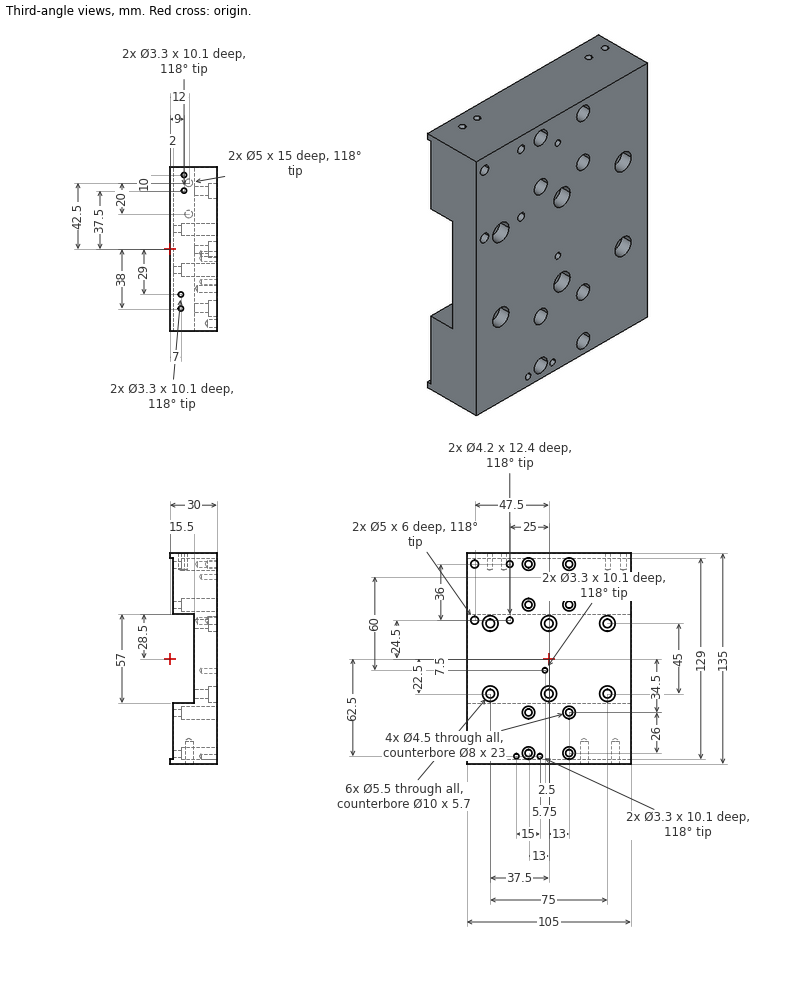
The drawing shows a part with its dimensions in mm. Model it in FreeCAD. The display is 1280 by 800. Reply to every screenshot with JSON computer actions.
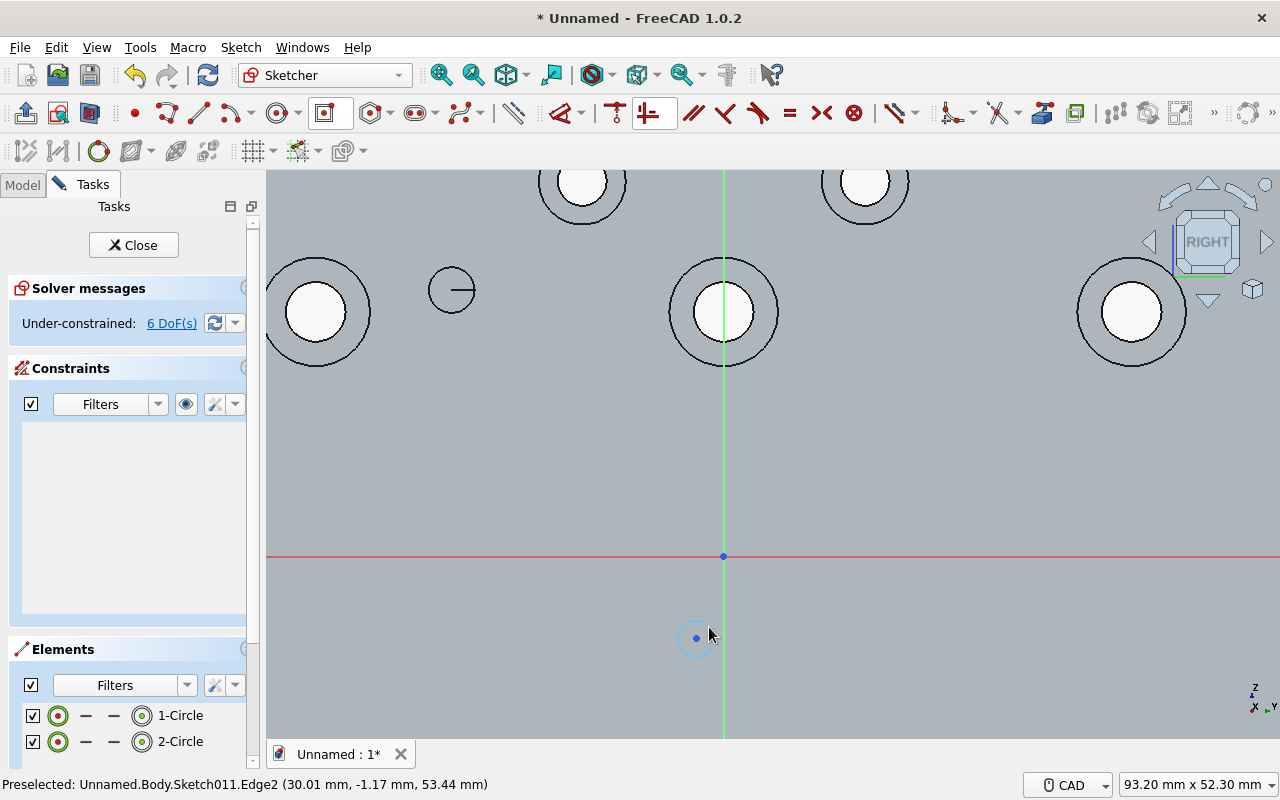
{"action": "left_click", "coordinate": [709, 626]}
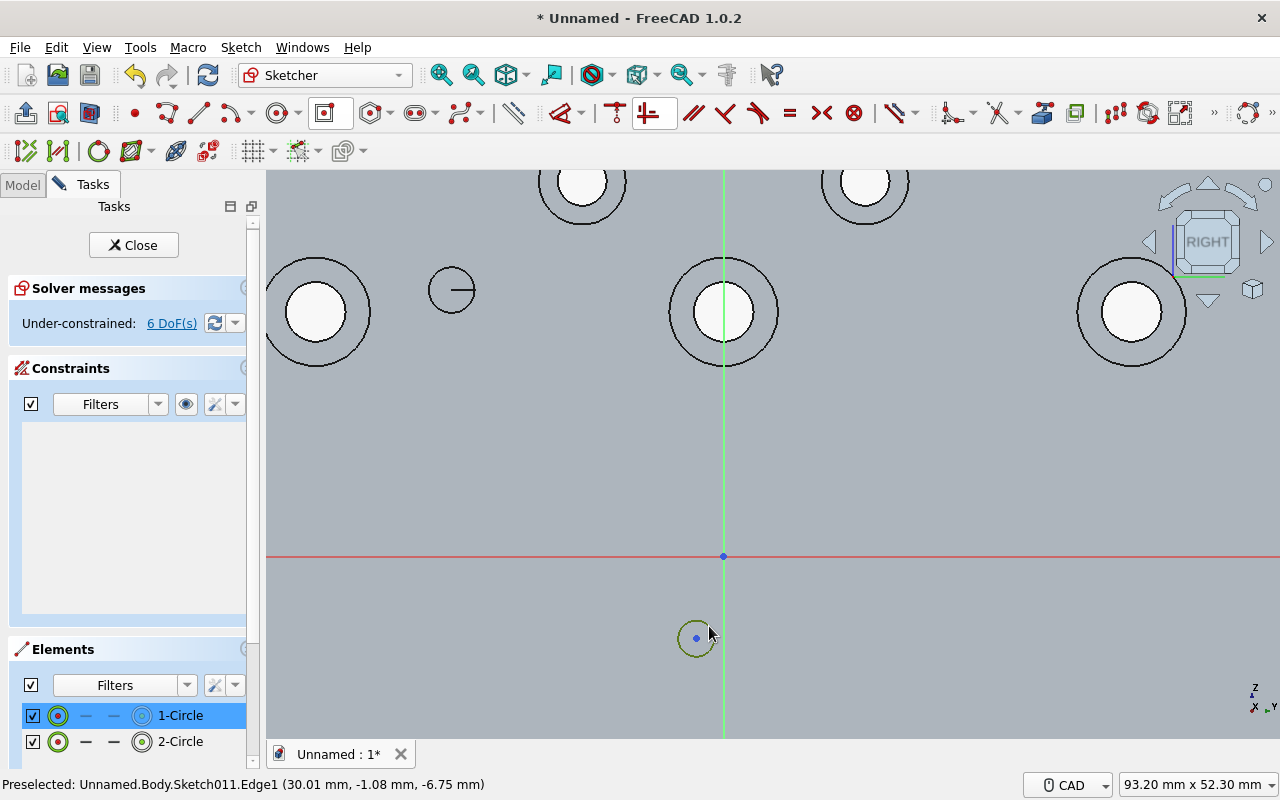
{"action": "scroll", "coordinate": [709, 628], "scroll_direction": "down", "scroll_amount": 3}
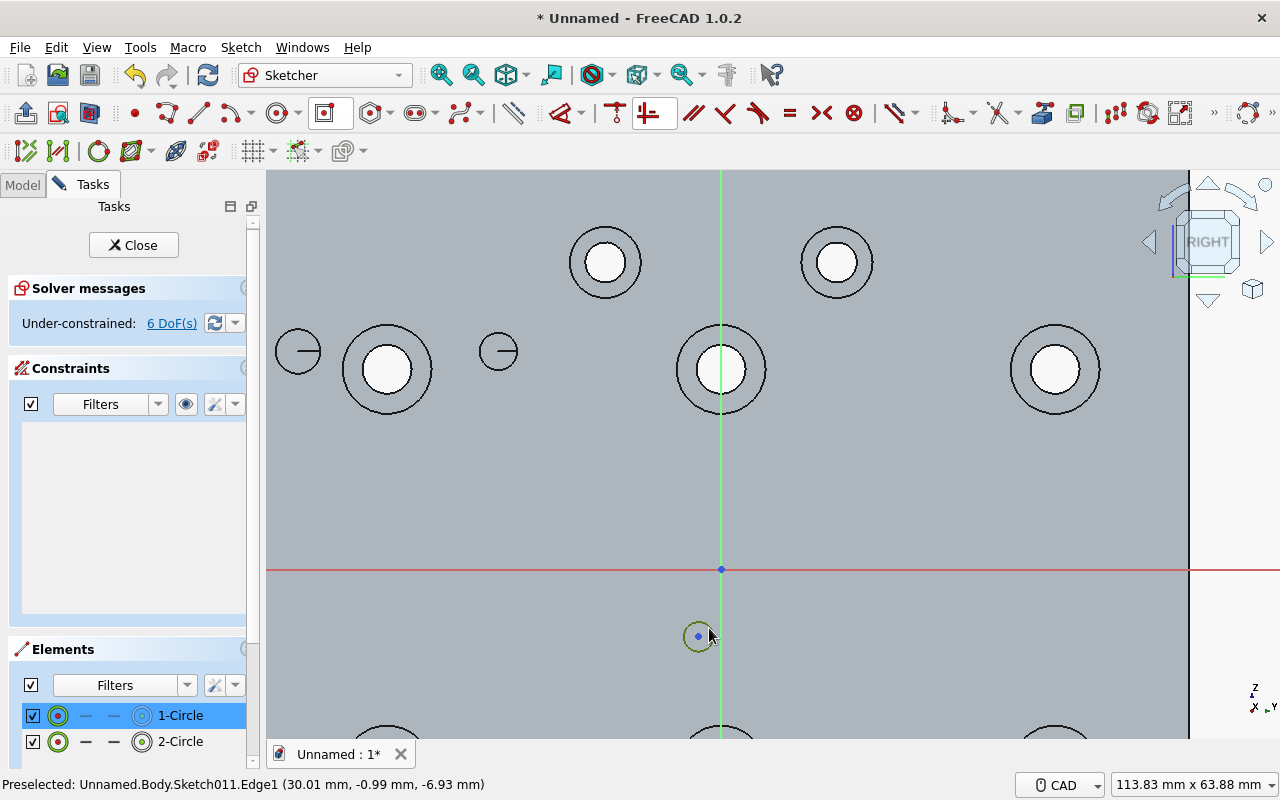
{"action": "scroll", "coordinate": [709, 269], "scroll_direction": "up", "scroll_amount": 3}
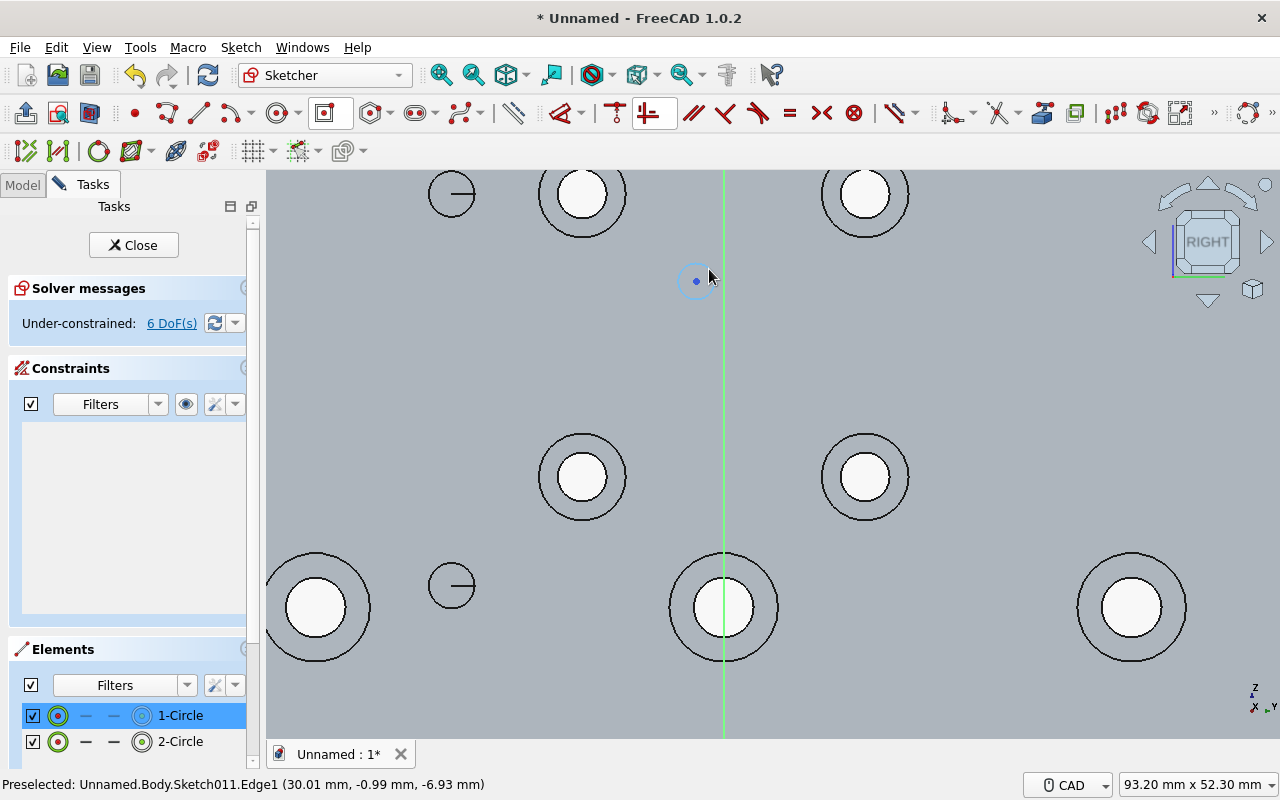
{"action": "left_click", "coordinate": [709, 269]}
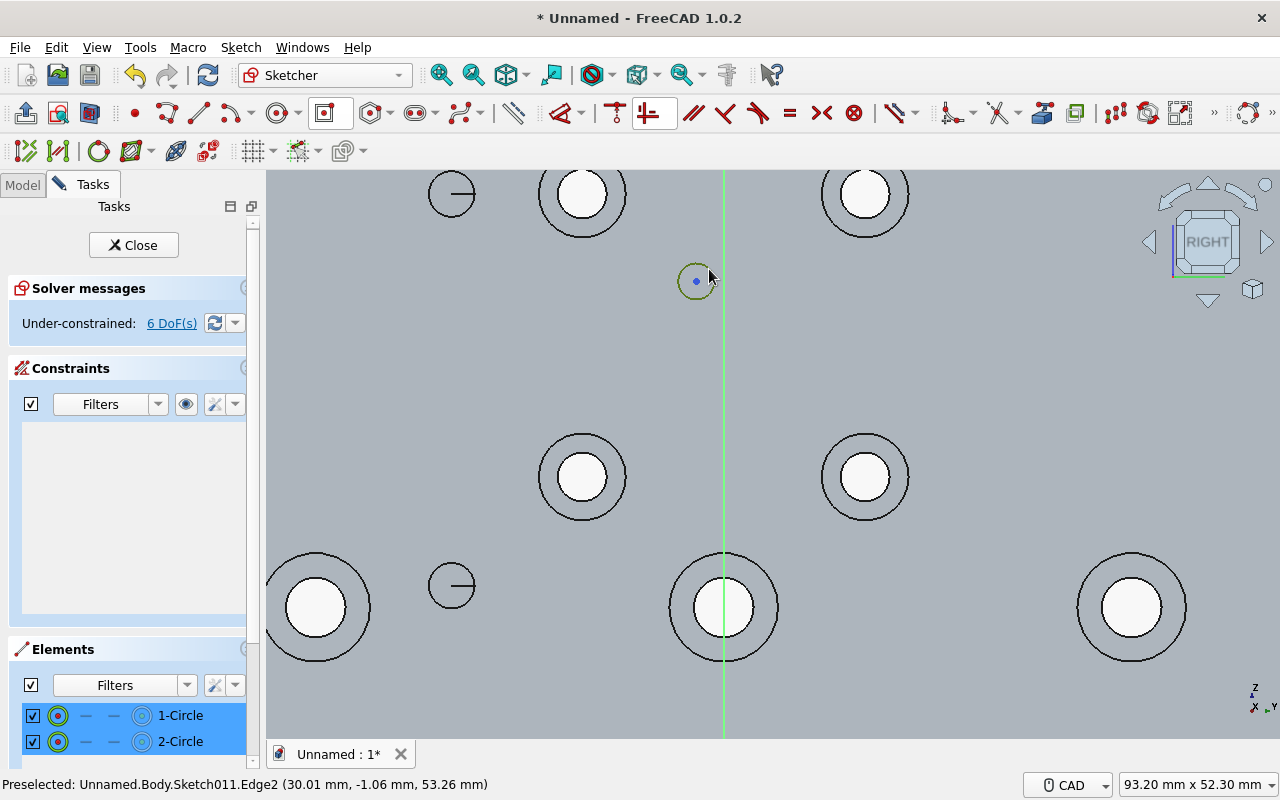
{"action": "left_click", "coordinate": [790, 114]}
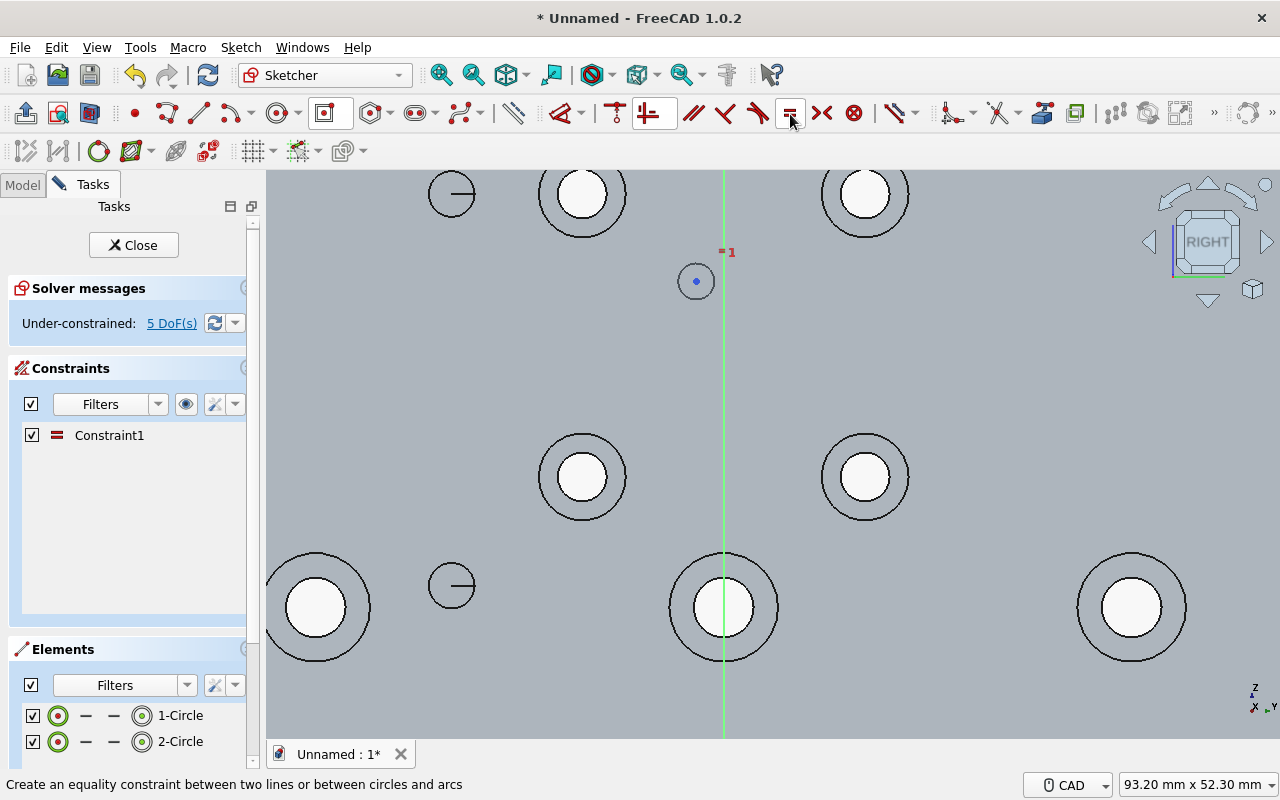
{"action": "scroll", "coordinate": [709, 268], "scroll_direction": "down", "scroll_amount": 3}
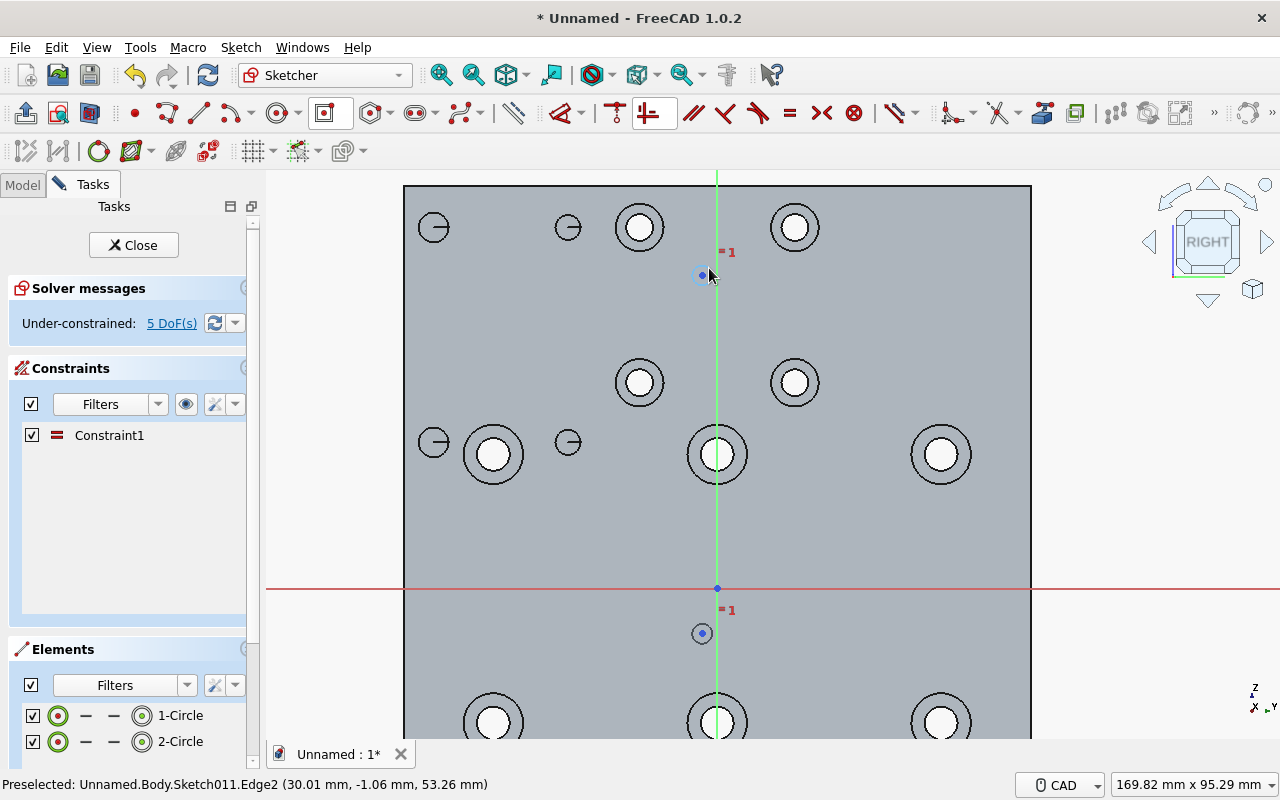
{"action": "left_click", "coordinate": [702, 634]}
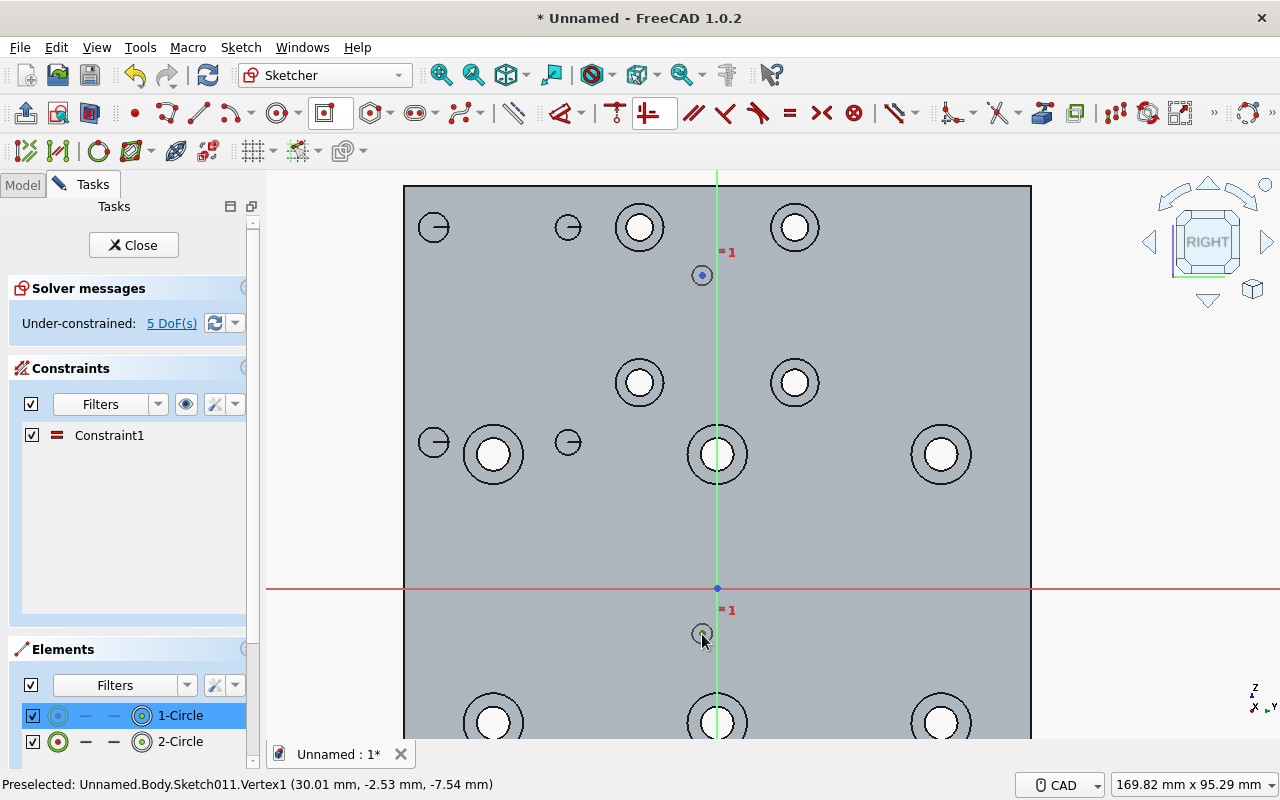
{"action": "left_click", "coordinate": [702, 275]}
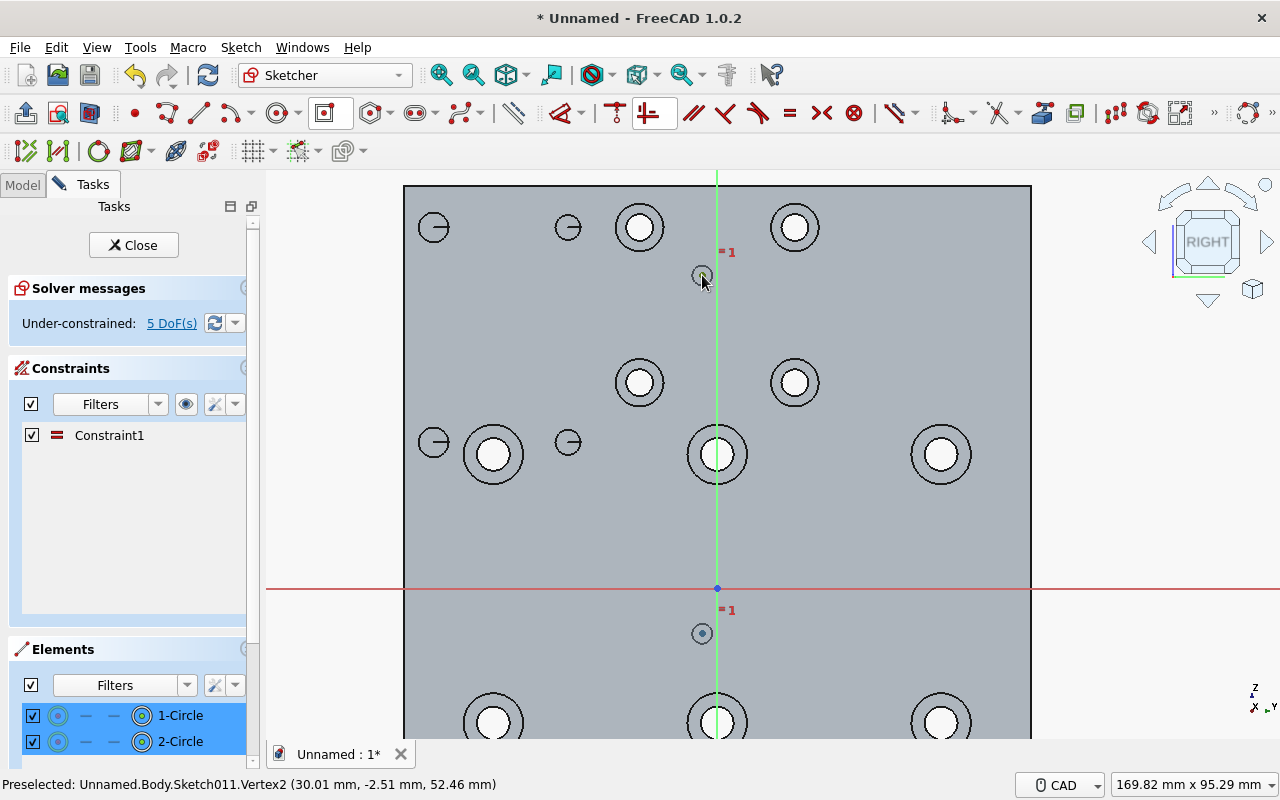
{"action": "left_click", "coordinate": [672, 114]}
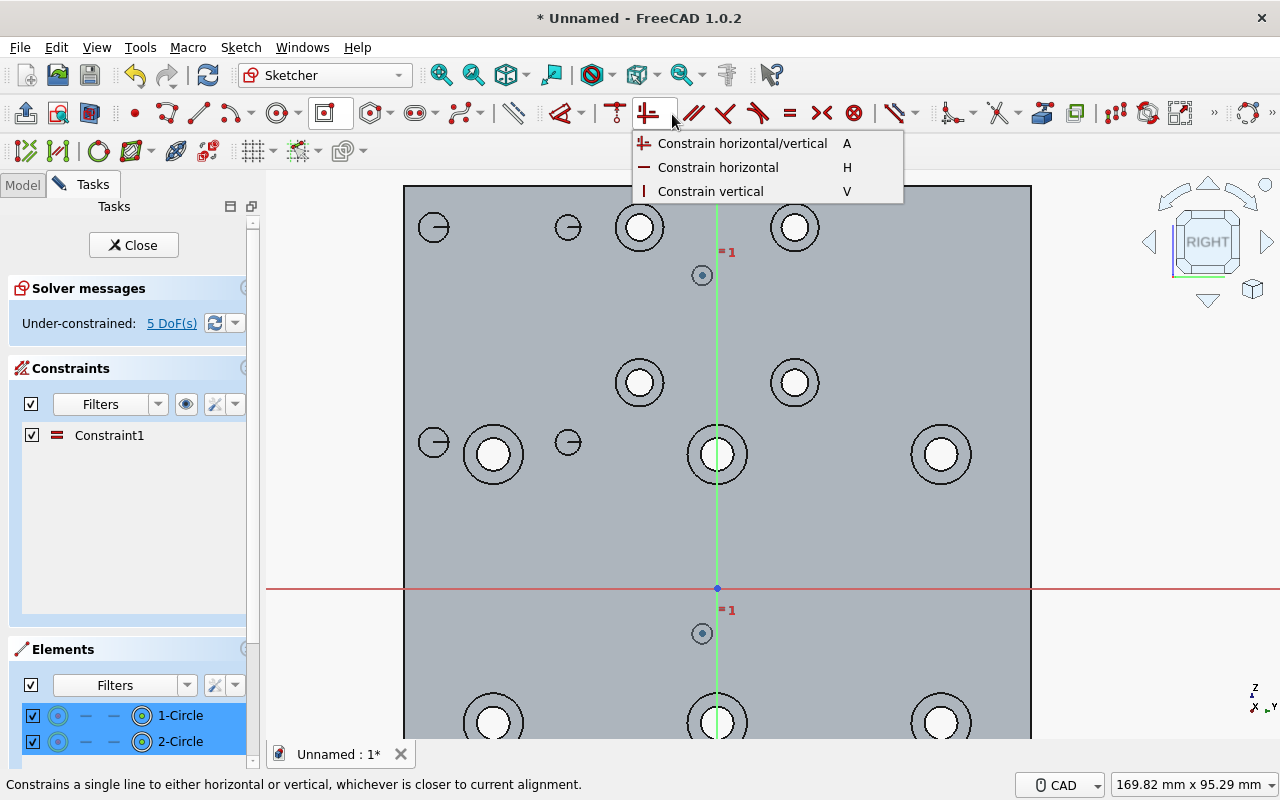
{"action": "left_click", "coordinate": [768, 191]}